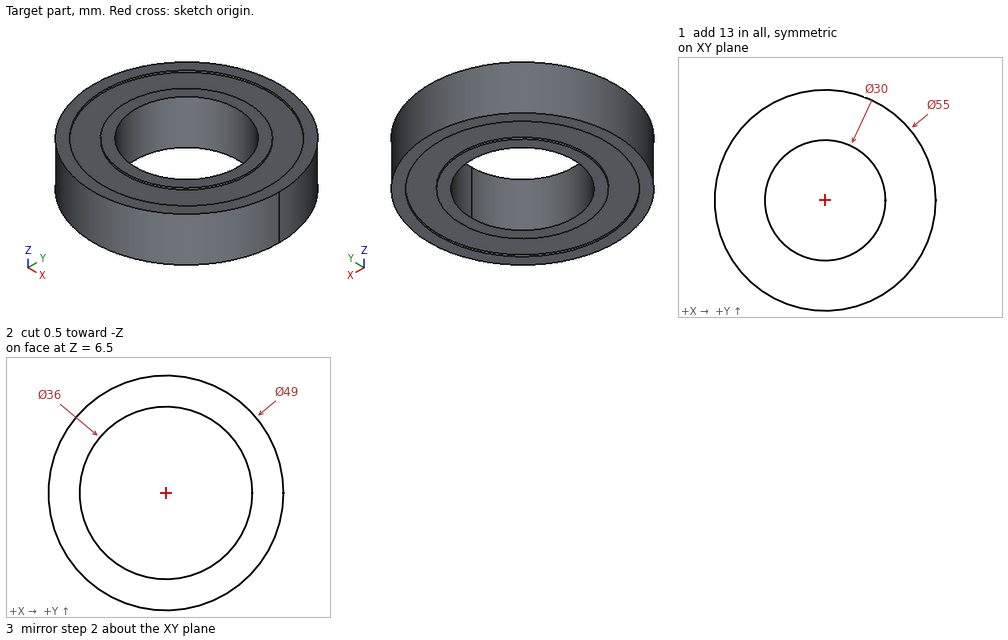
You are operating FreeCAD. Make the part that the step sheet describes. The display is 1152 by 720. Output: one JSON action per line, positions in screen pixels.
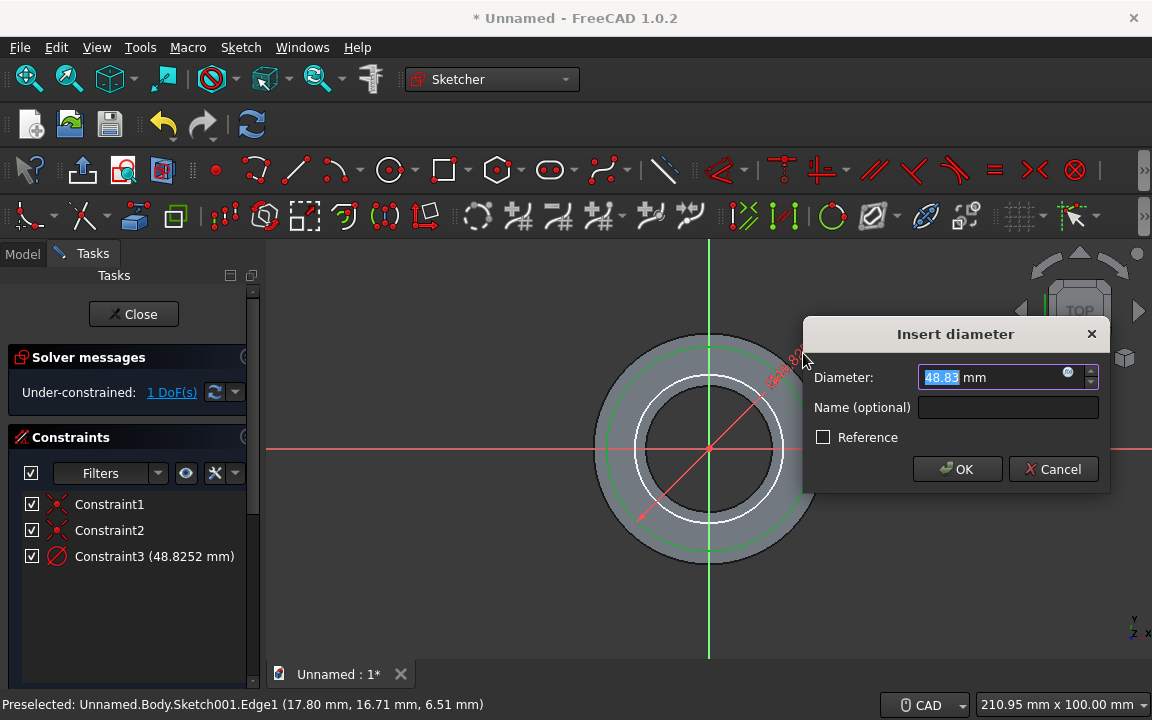
{"action": "type", "text": "49"}
{"action": "key", "text": "Return"}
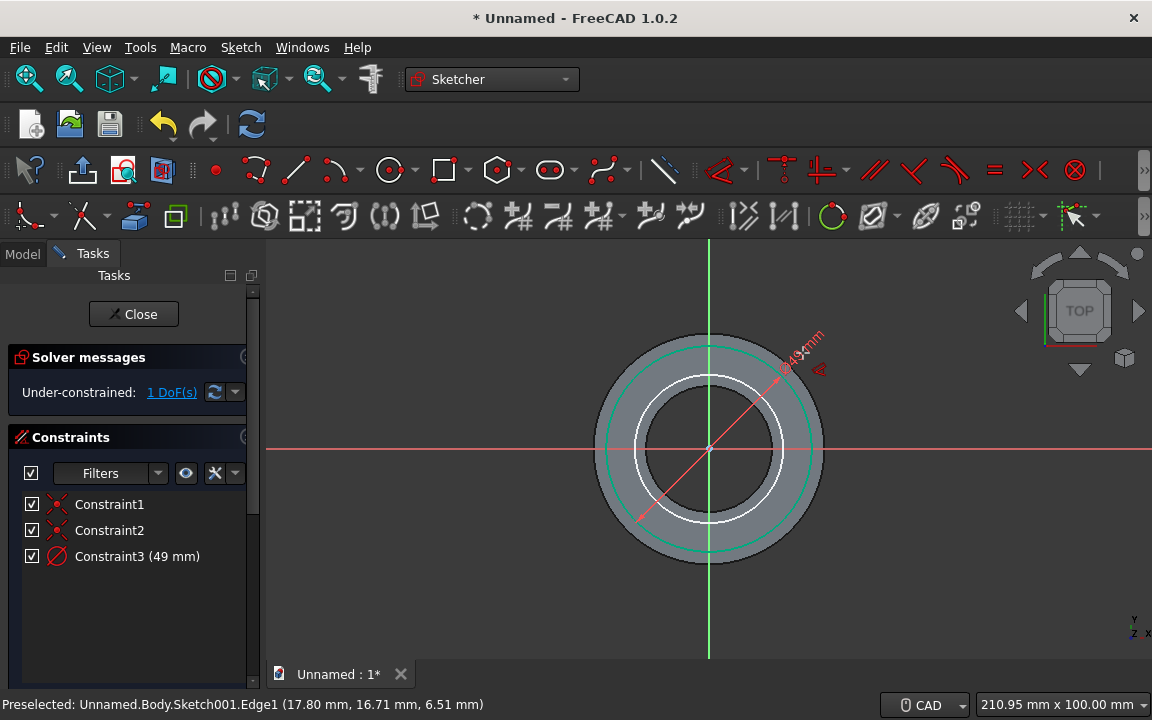
{"action": "left_click", "coordinate": [761, 396]}
{"action": "left_click", "coordinate": [833, 411]}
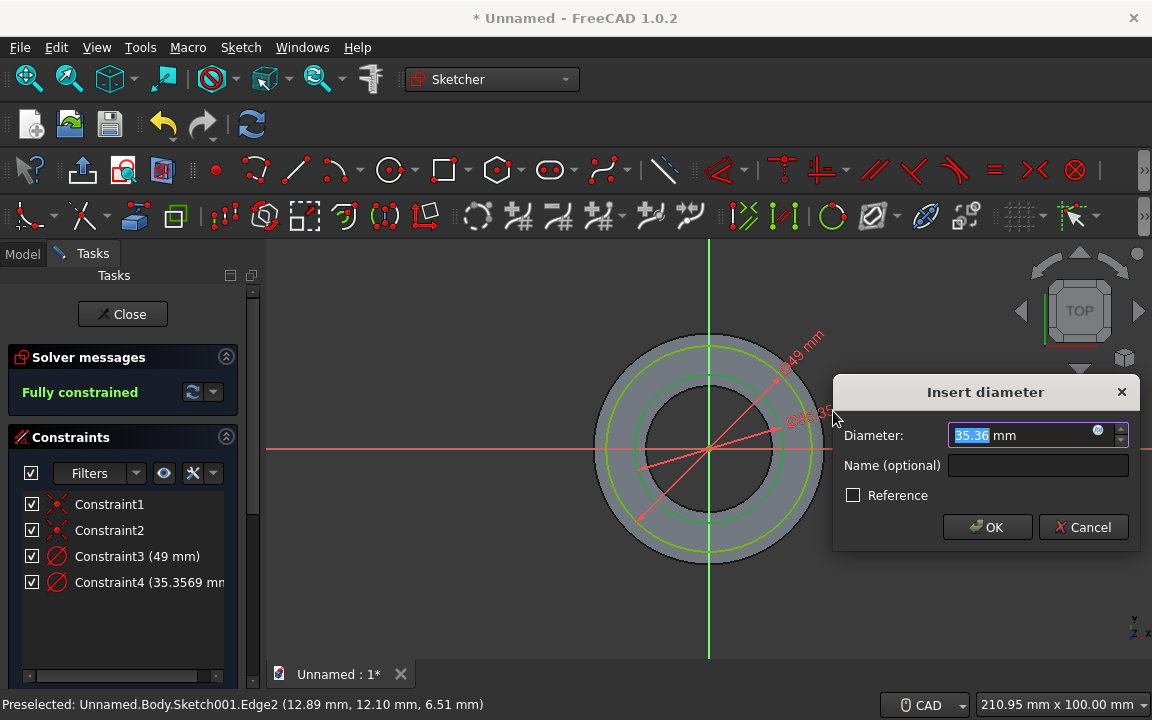
{"action": "type", "text": "36"}
{"action": "key", "text": "Return"}
{"action": "key", "text": "Escape"}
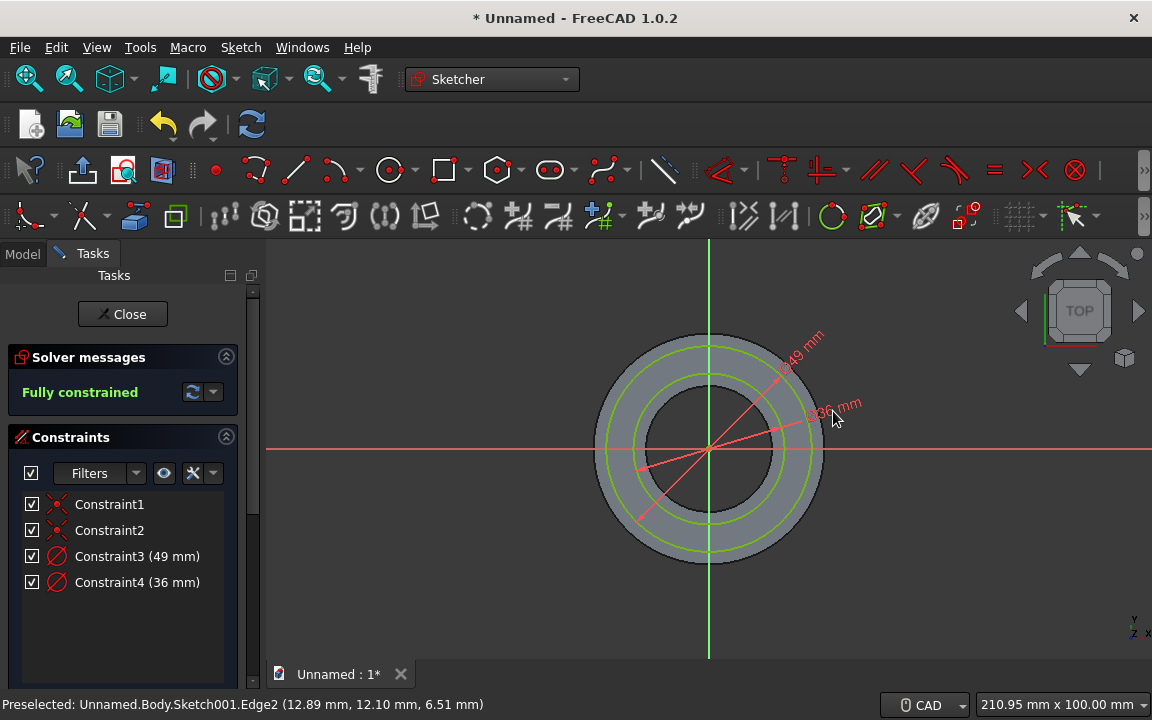
{"action": "left_click", "coordinate": [123, 314]}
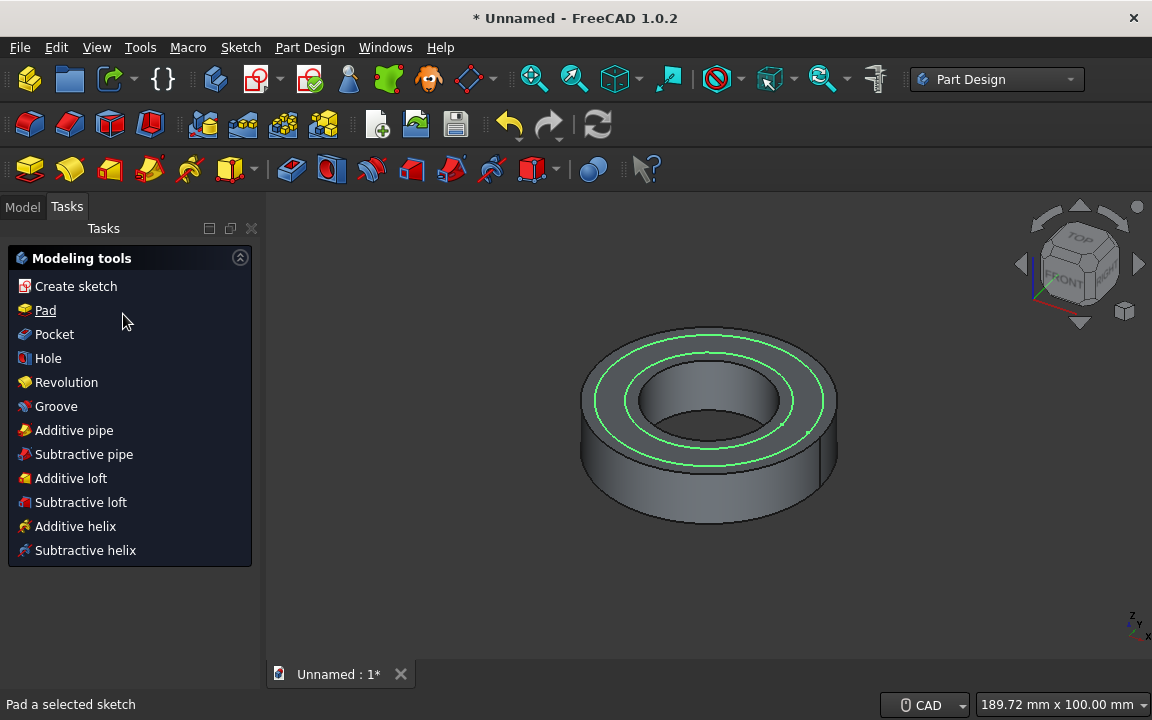
{"action": "left_click", "coordinate": [292, 170]}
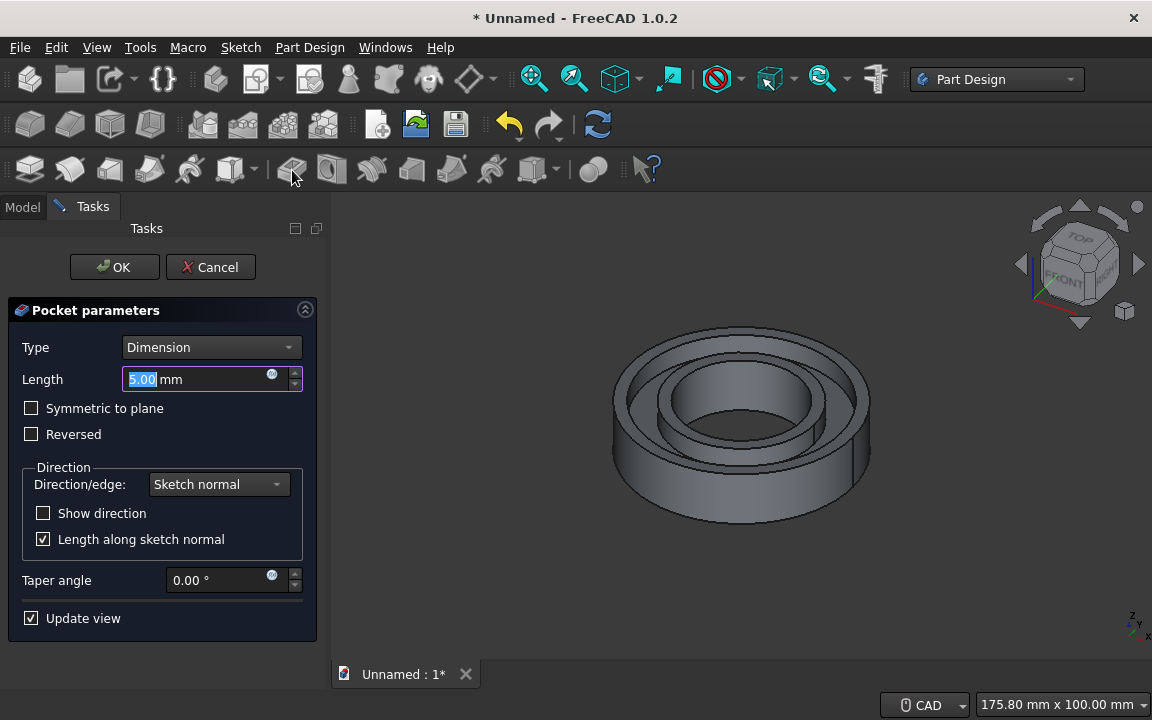
{"action": "type", "text": "0.5"}
{"action": "key", "text": "Tab"}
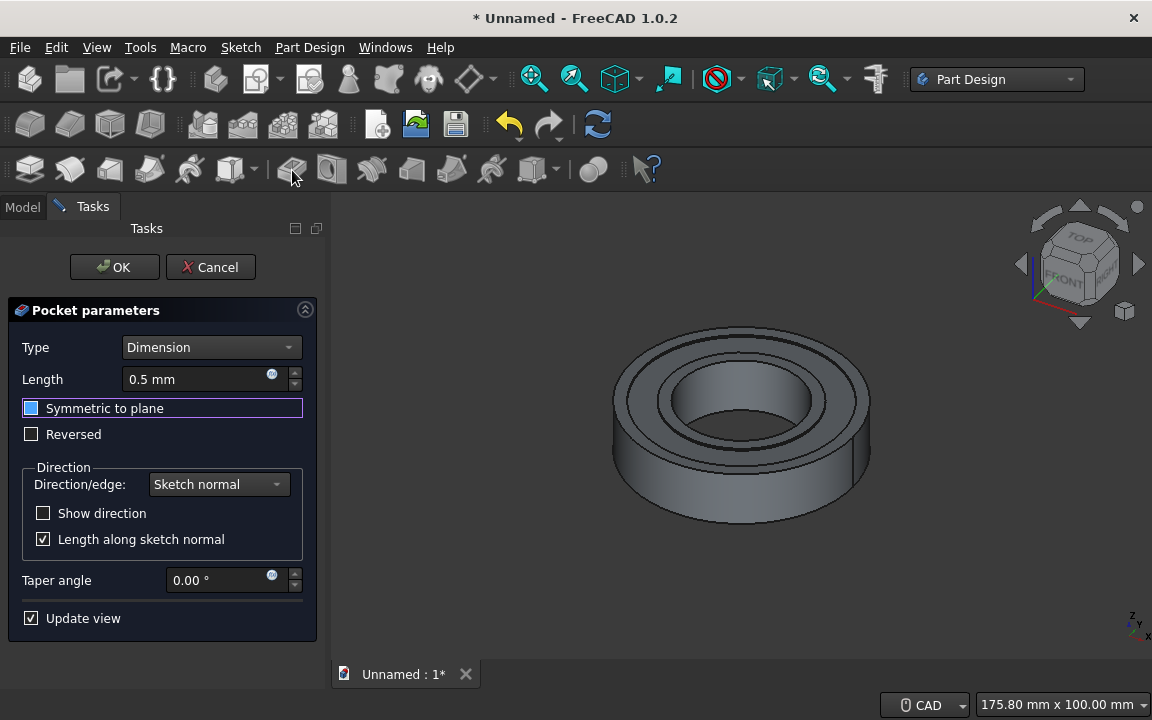
{"action": "left_click", "coordinate": [115, 267]}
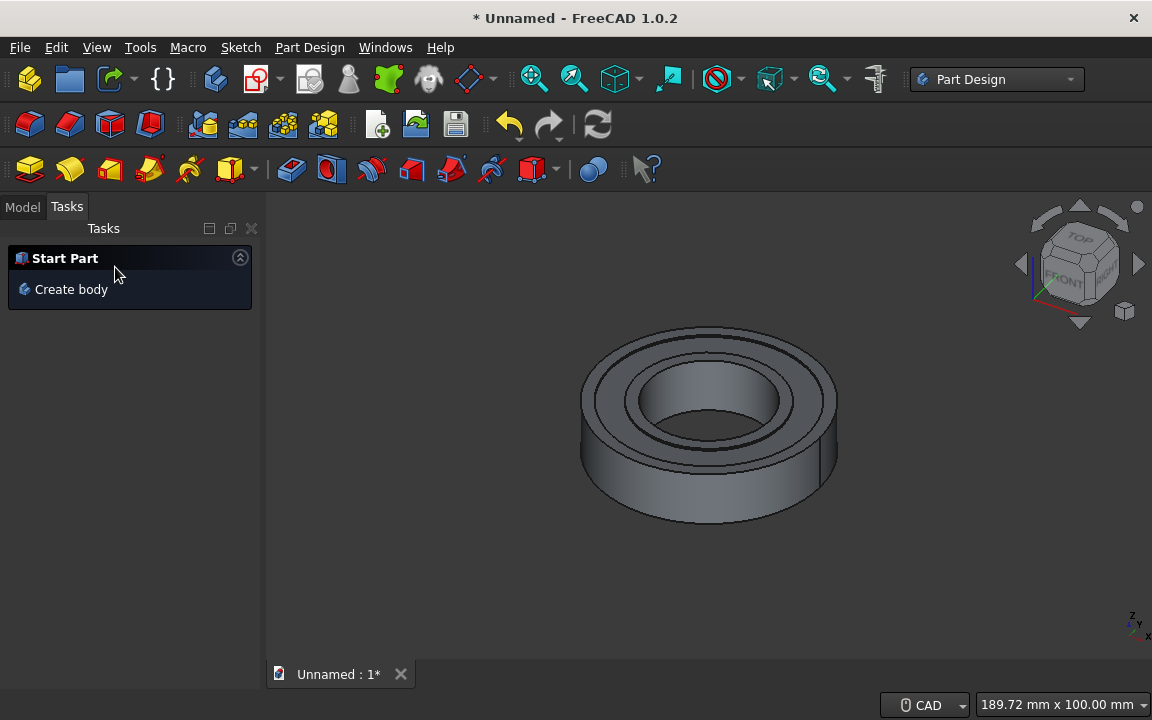
{"action": "left_click", "coordinate": [23, 206]}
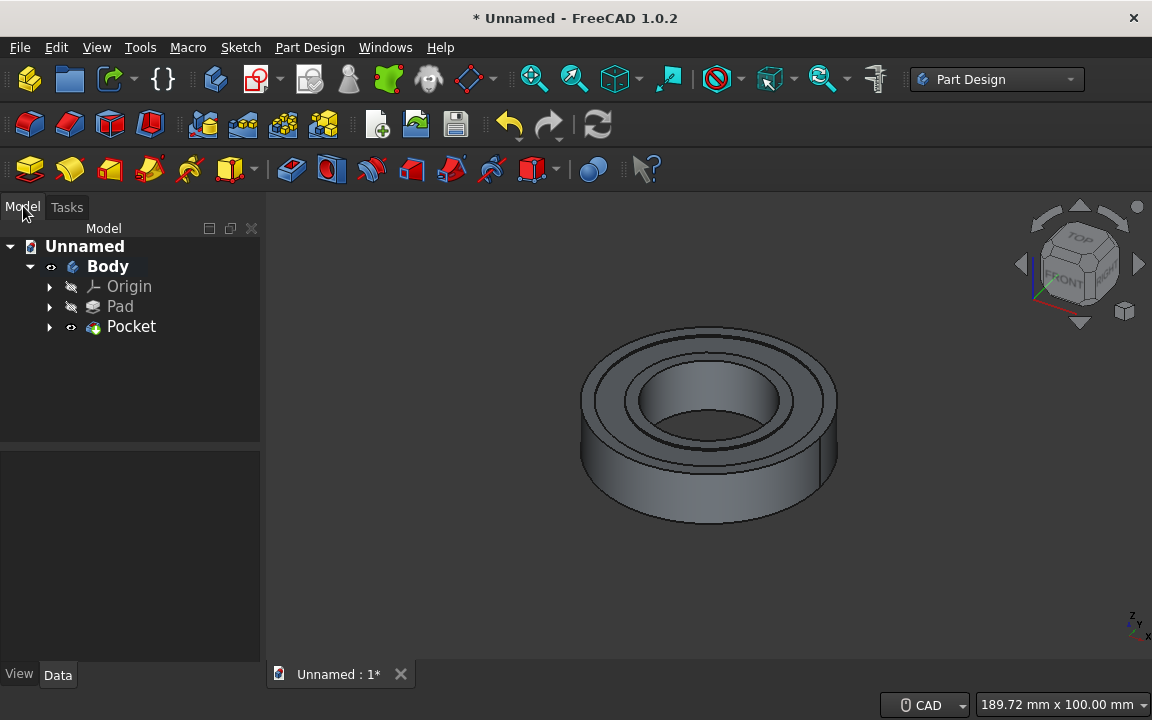
{"action": "left_click", "coordinate": [116, 327]}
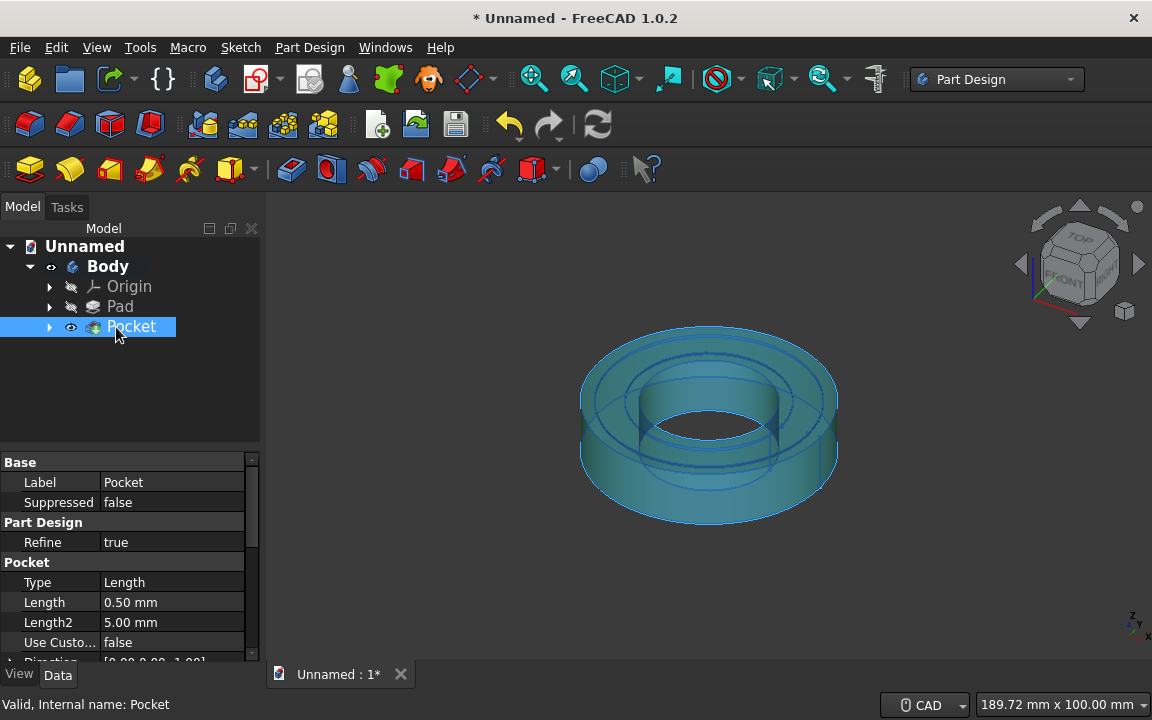
{"action": "left_click", "coordinate": [204, 124]}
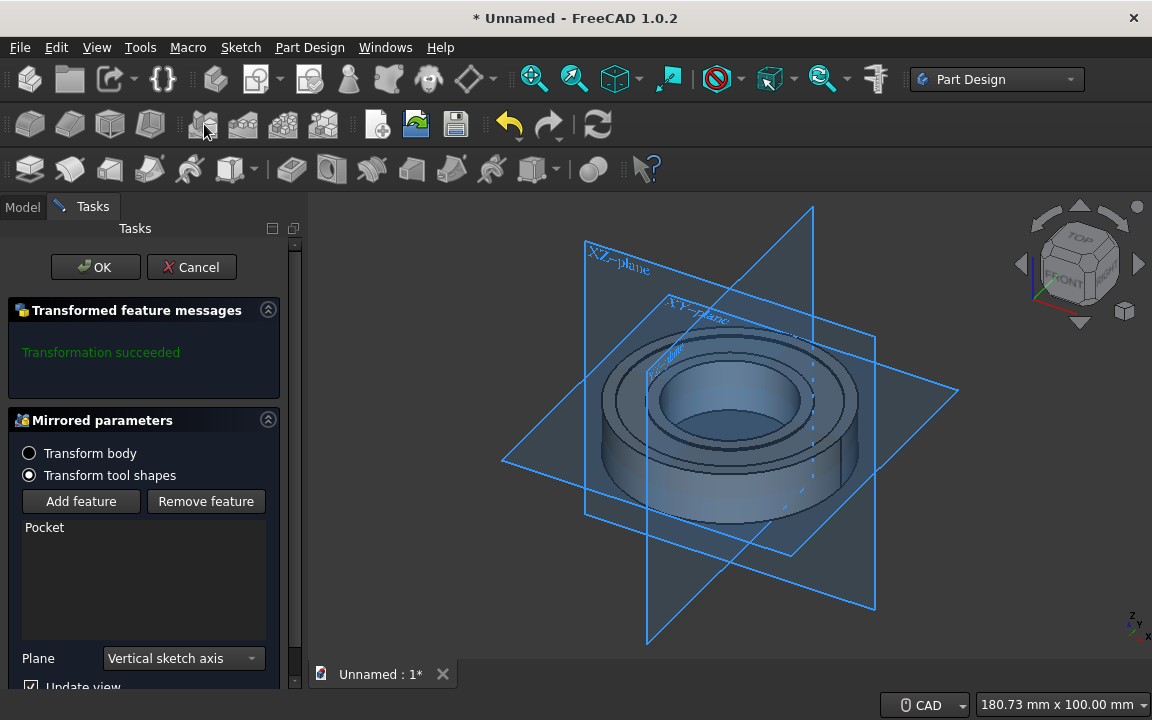
{"action": "left_click", "coordinate": [184, 658]}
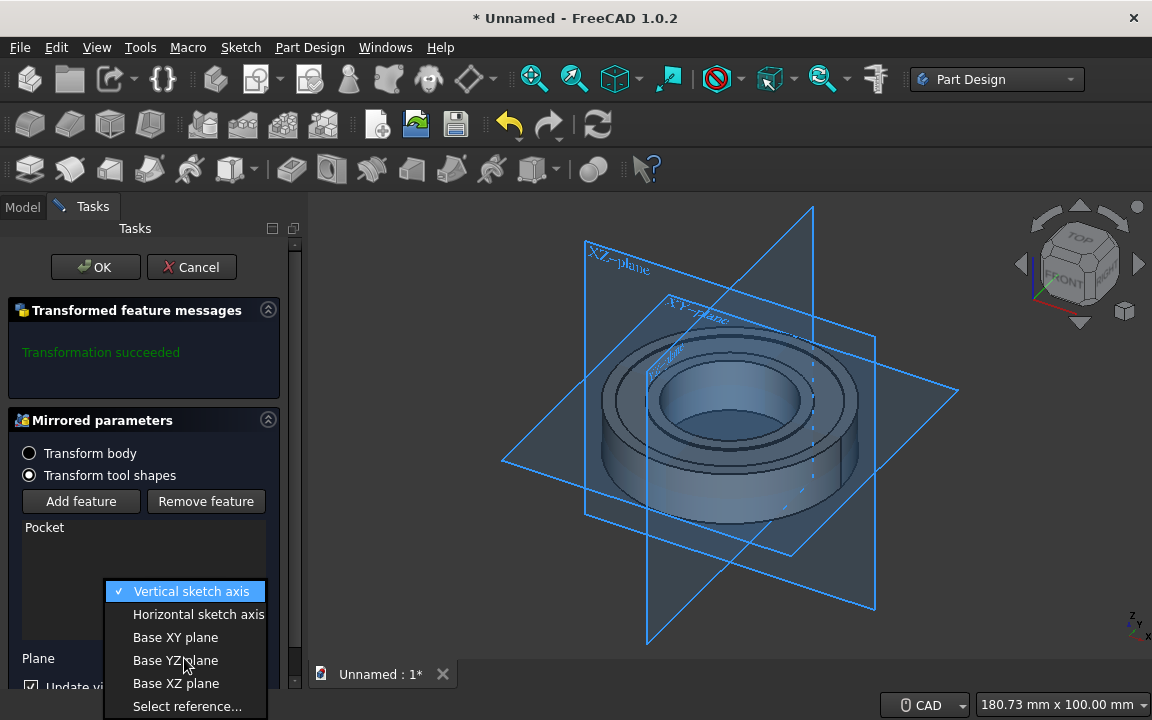
{"action": "left_click", "coordinate": [184, 638]}